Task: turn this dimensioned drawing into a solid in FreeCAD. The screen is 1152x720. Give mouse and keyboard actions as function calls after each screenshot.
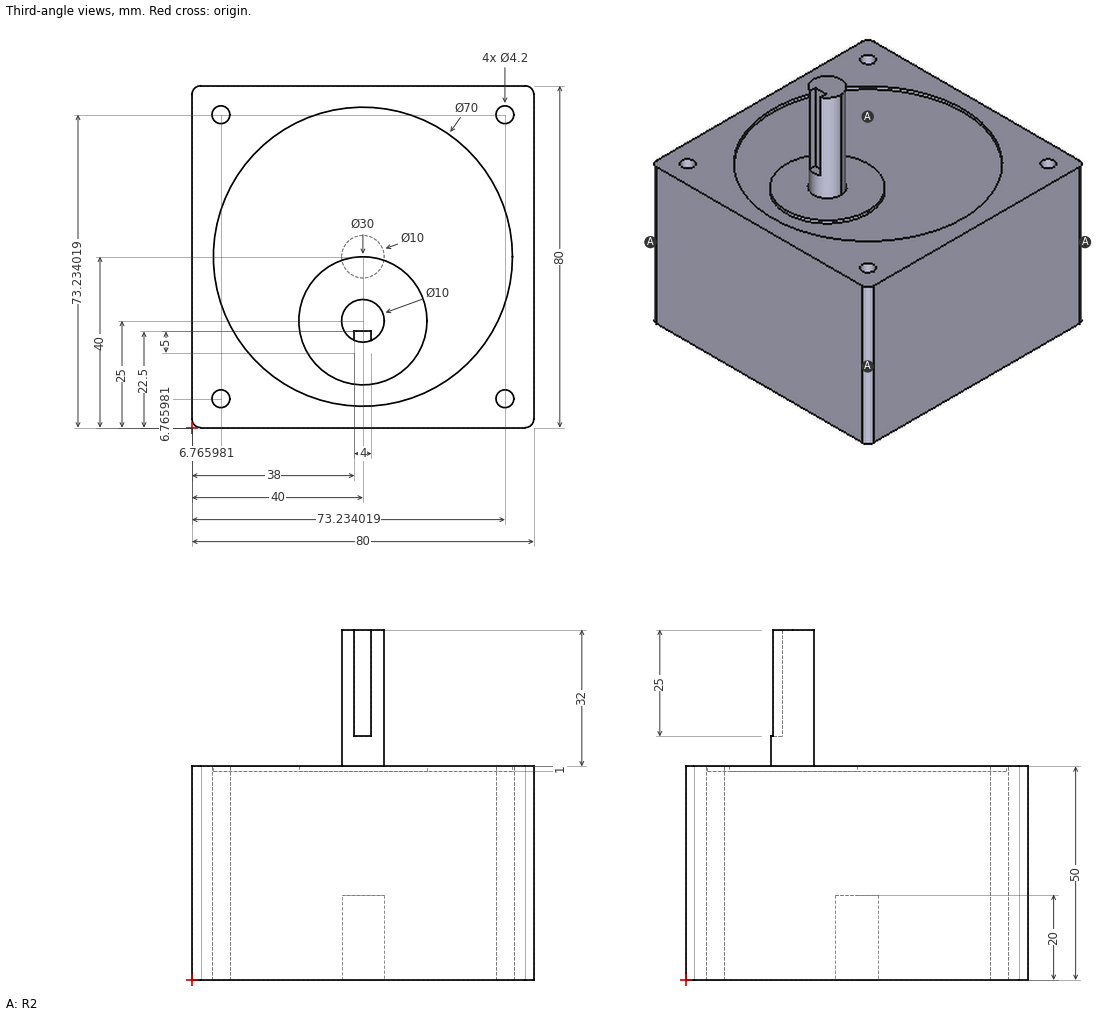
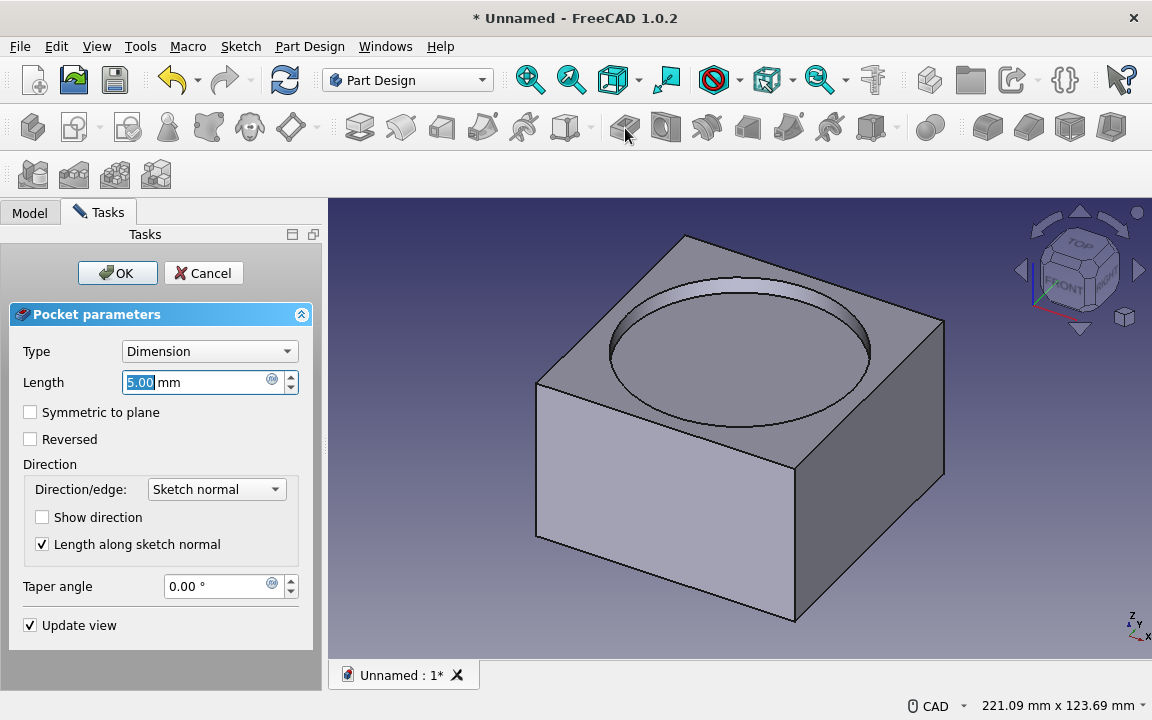
text(1)
key(Tab)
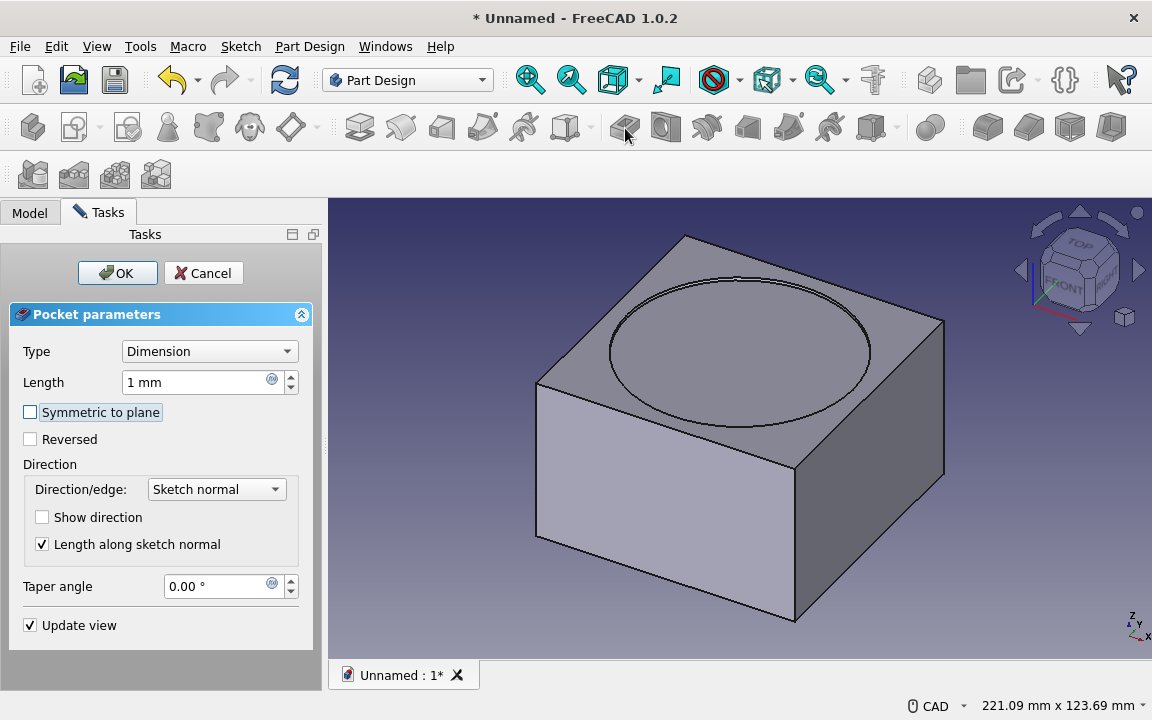
click(118, 273)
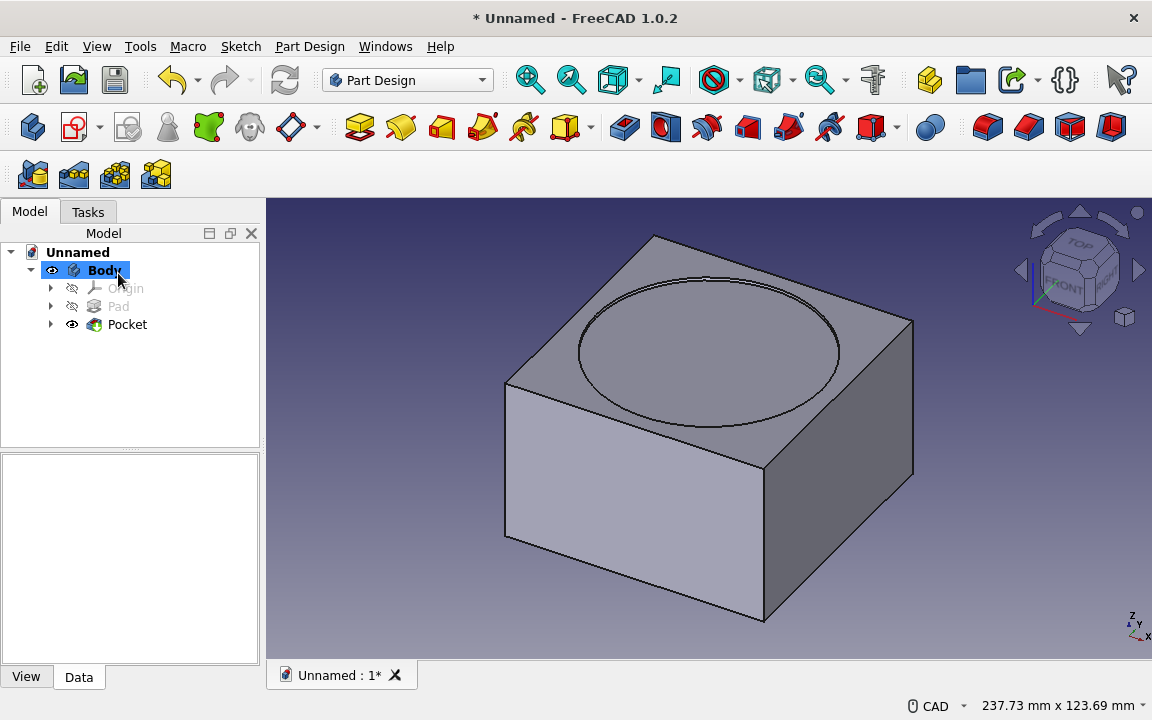
click(764, 544)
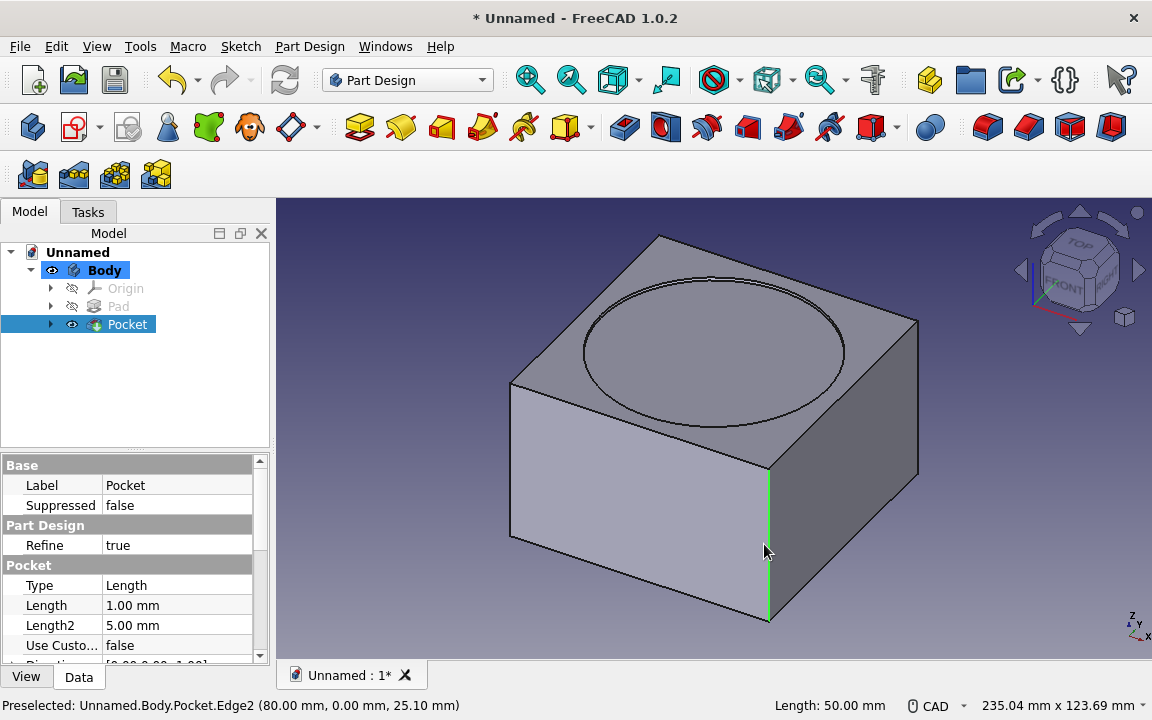
key(0)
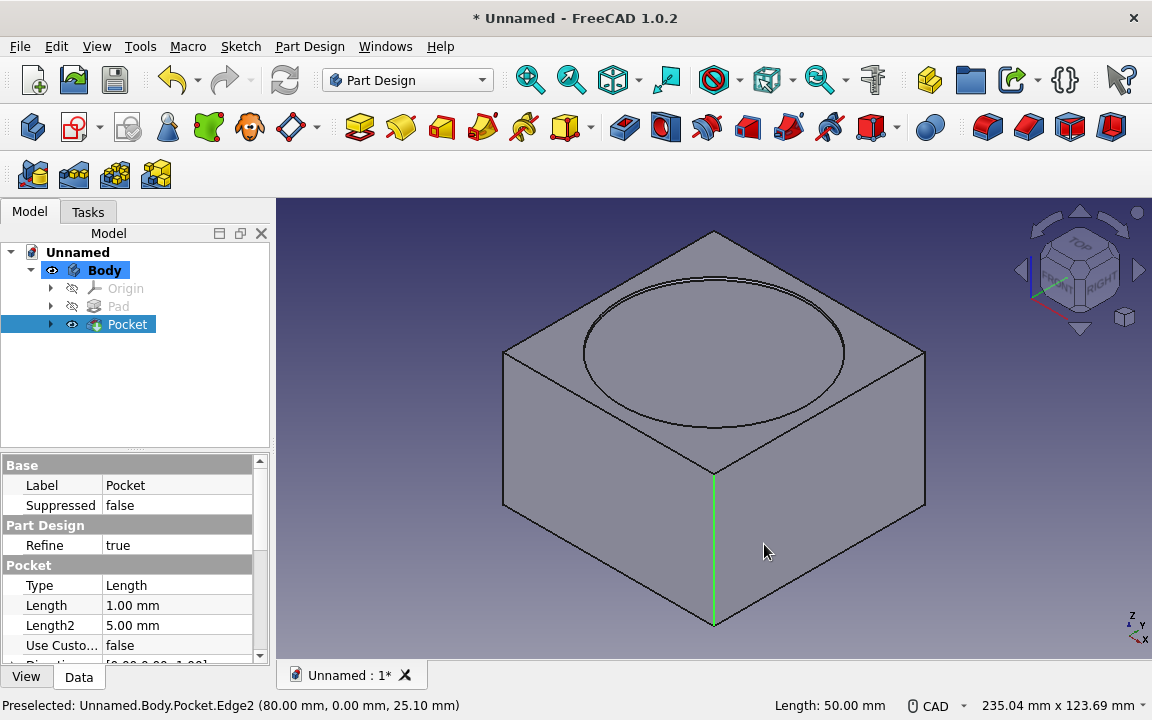
key(2)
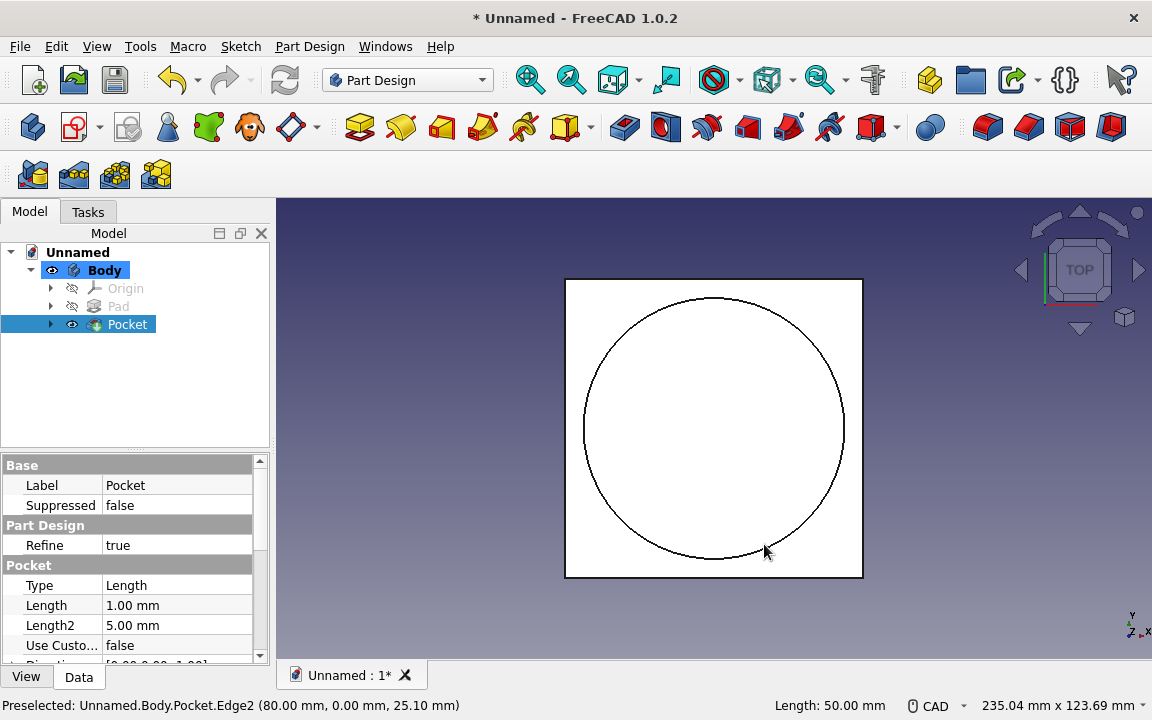
key(1)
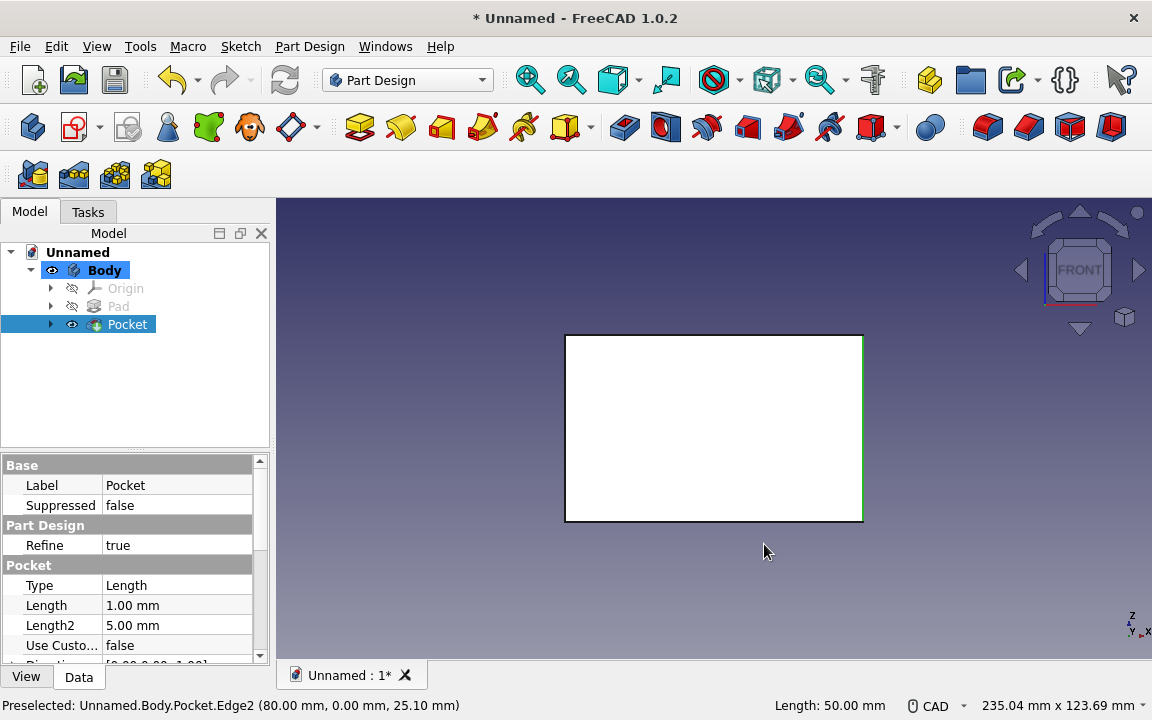
click(531, 80)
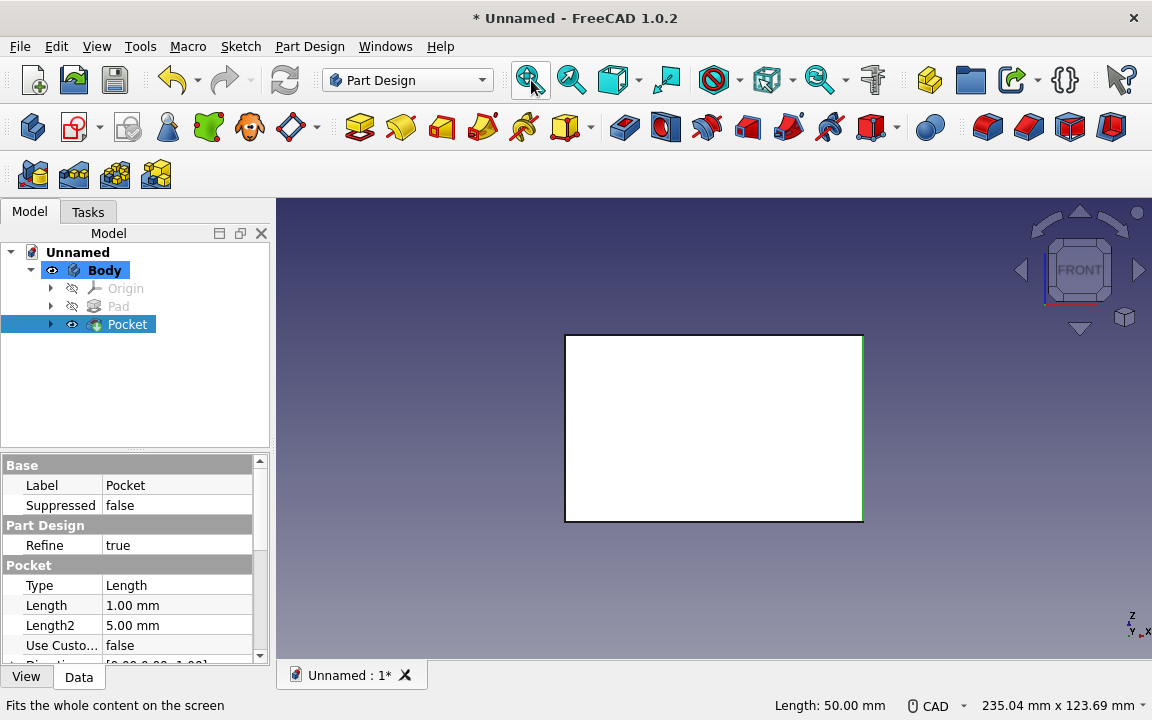
click(565, 428, ctrl)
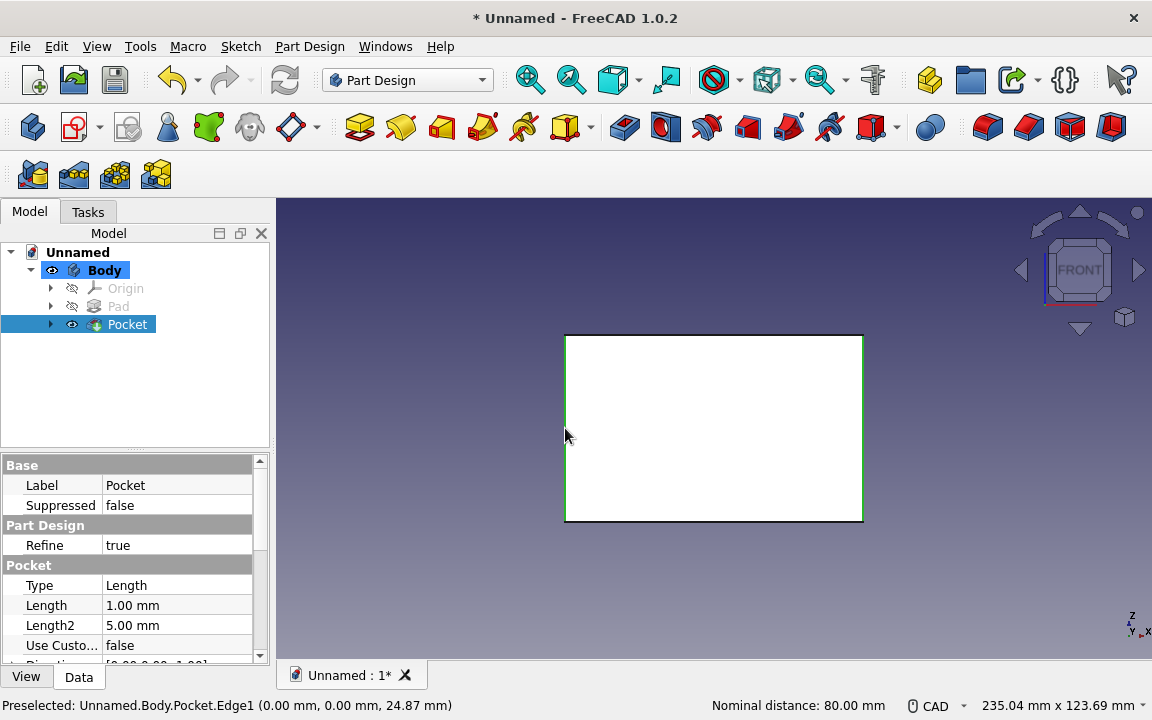
key(3)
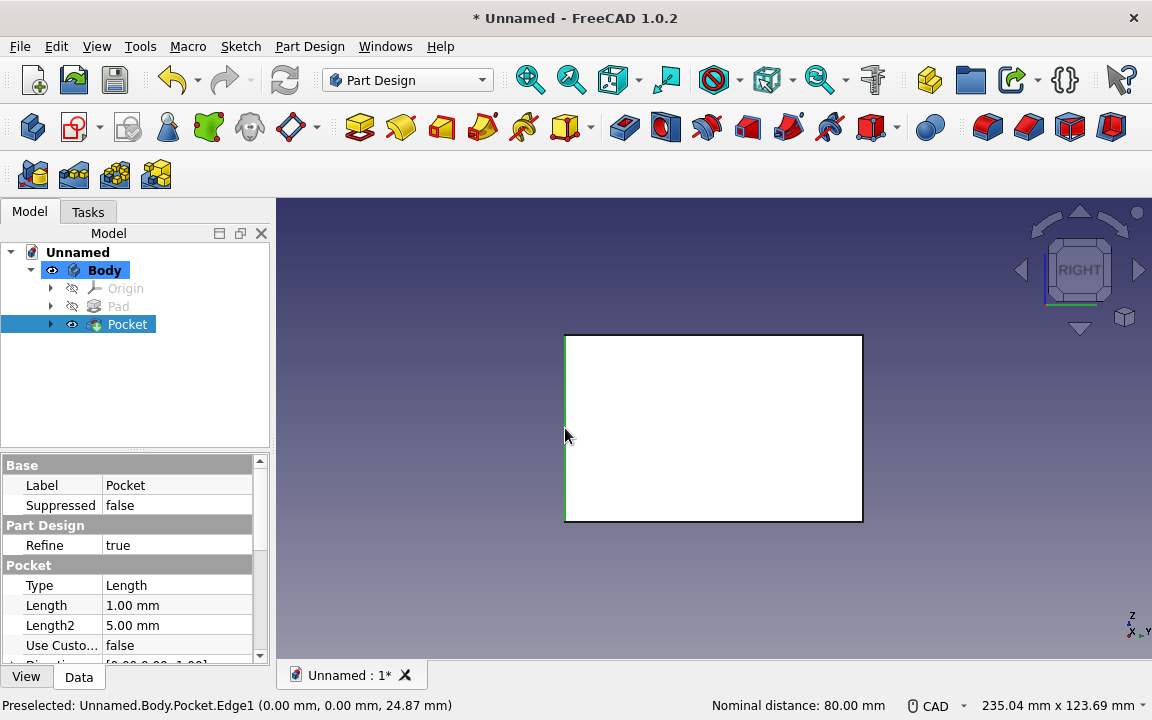
click(531, 80)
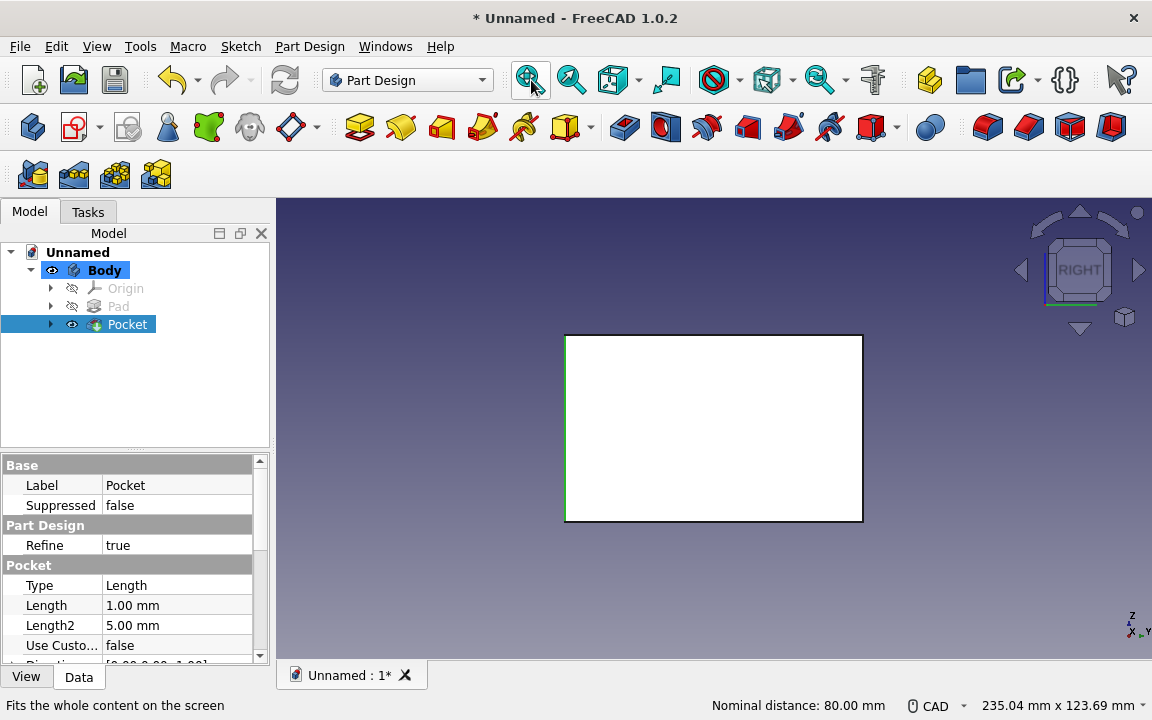
click(863, 427, ctrl)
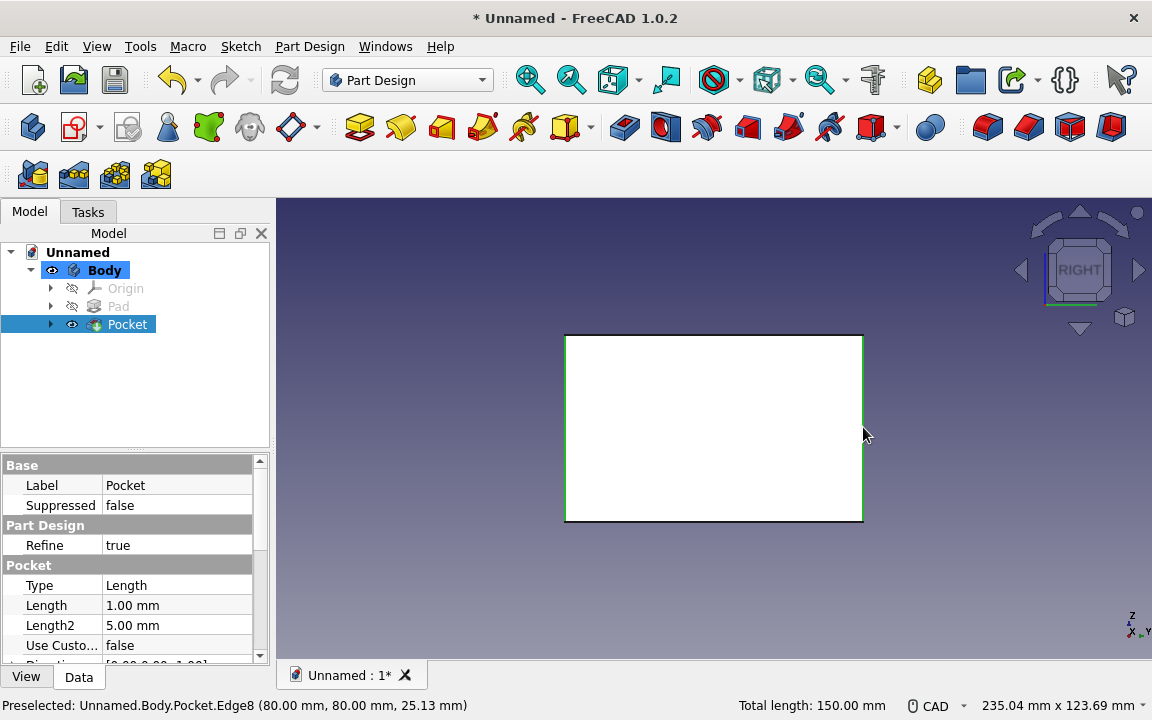
key(5)